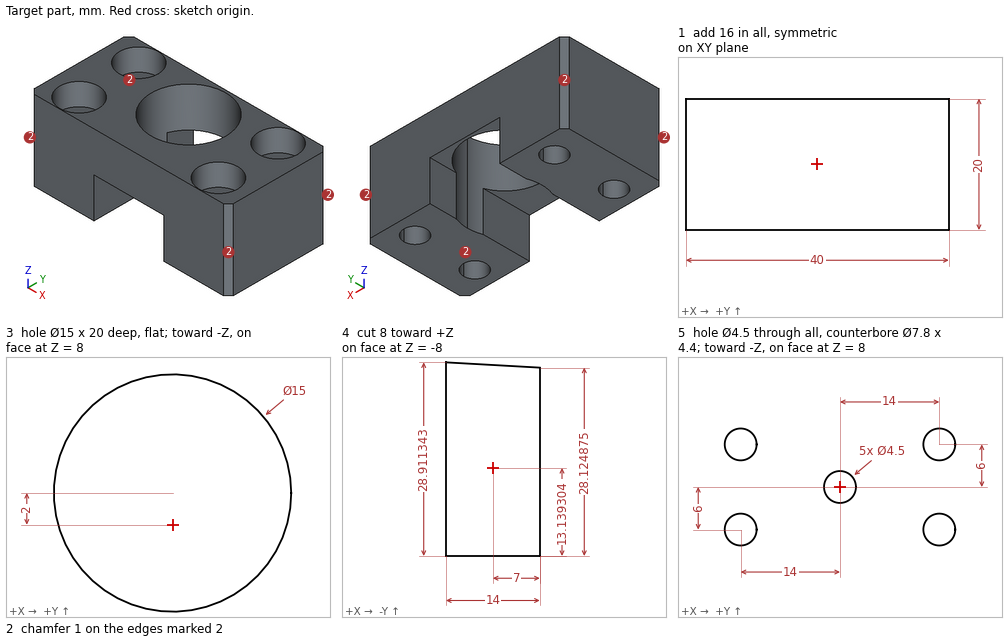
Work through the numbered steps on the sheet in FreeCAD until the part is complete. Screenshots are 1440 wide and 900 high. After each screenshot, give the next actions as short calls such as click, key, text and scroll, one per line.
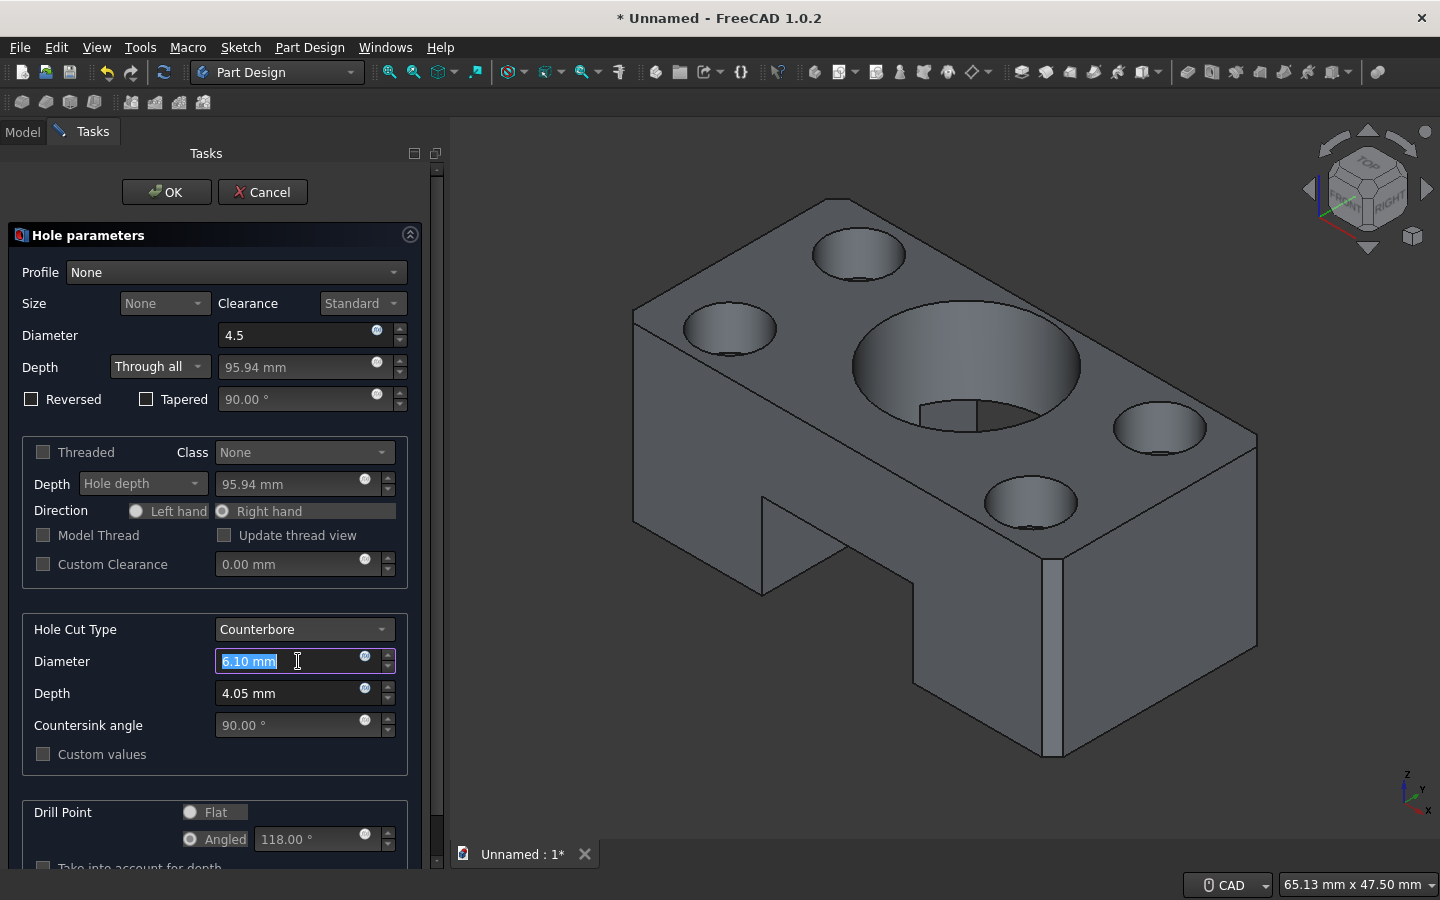
text(7.8)
key(Tab)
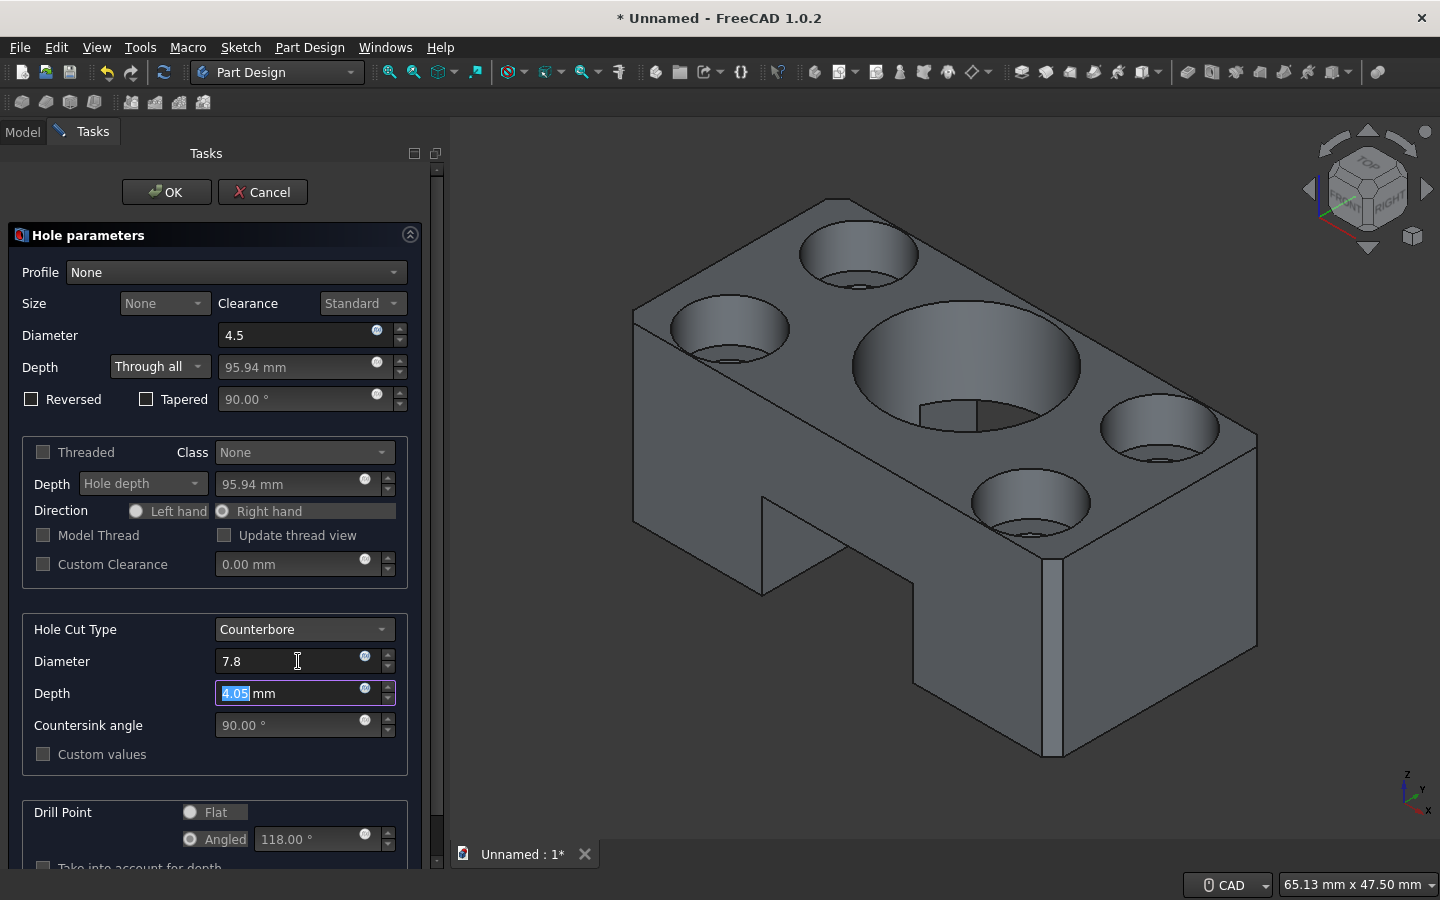
text(4.4)
key(Tab)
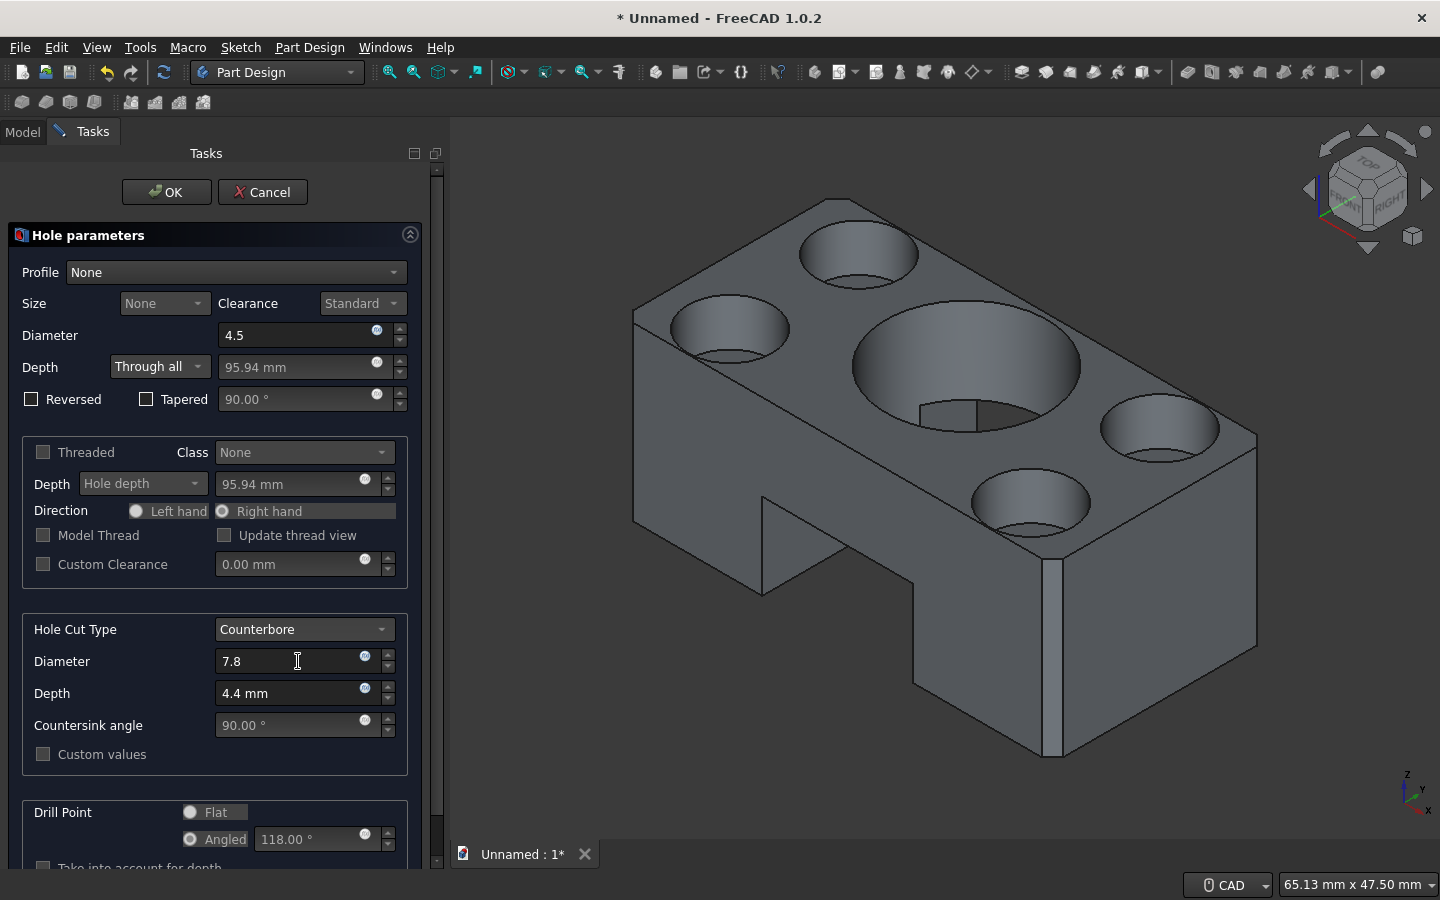
click(167, 192)